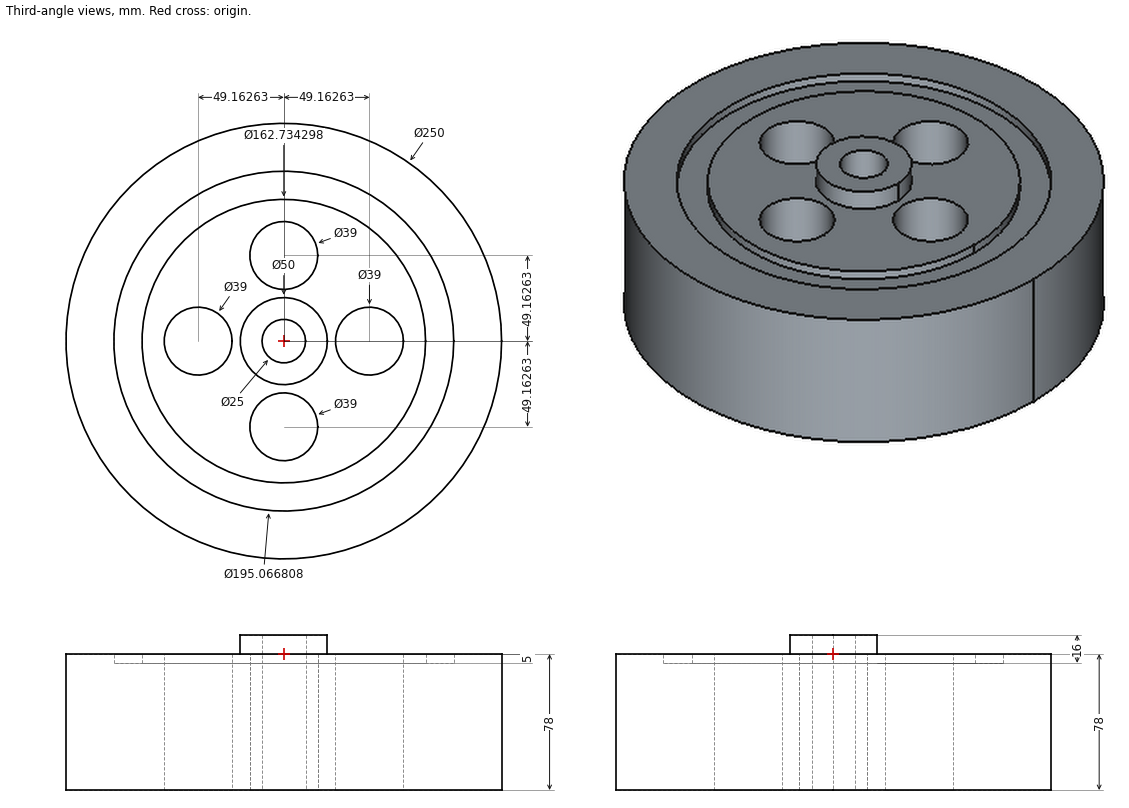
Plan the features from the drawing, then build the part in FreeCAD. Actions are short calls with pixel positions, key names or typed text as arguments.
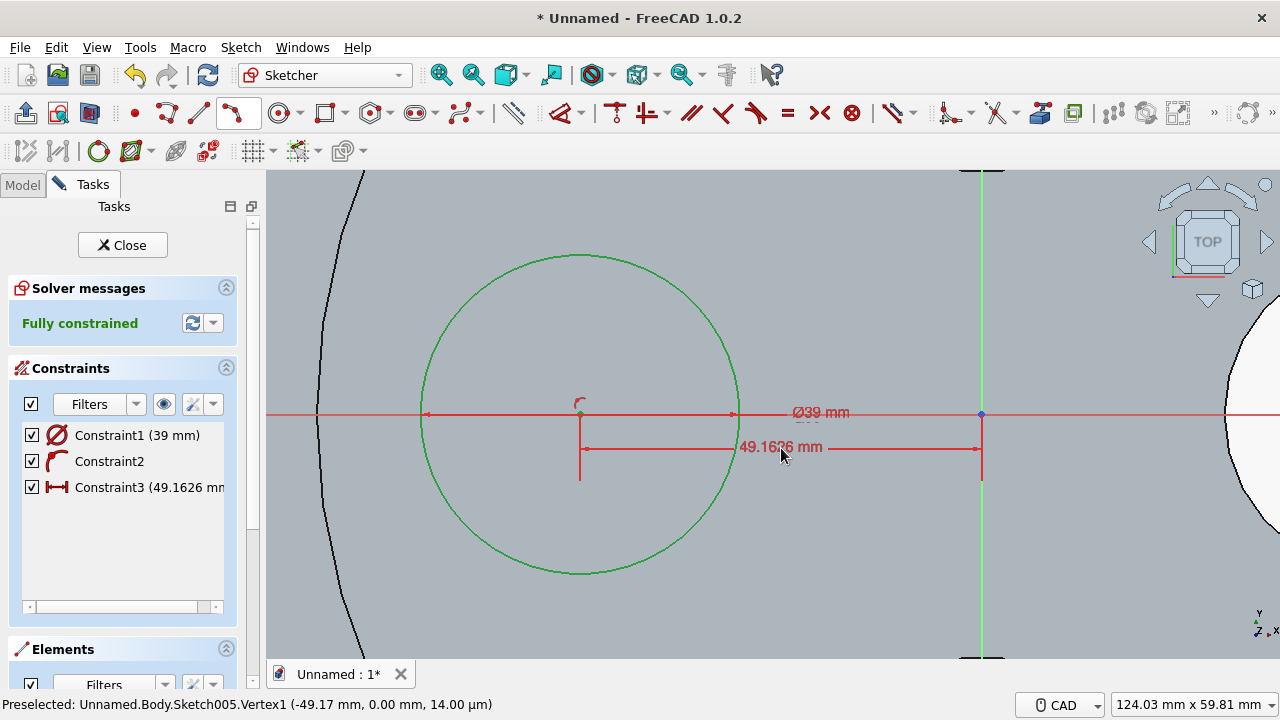
click(123, 245)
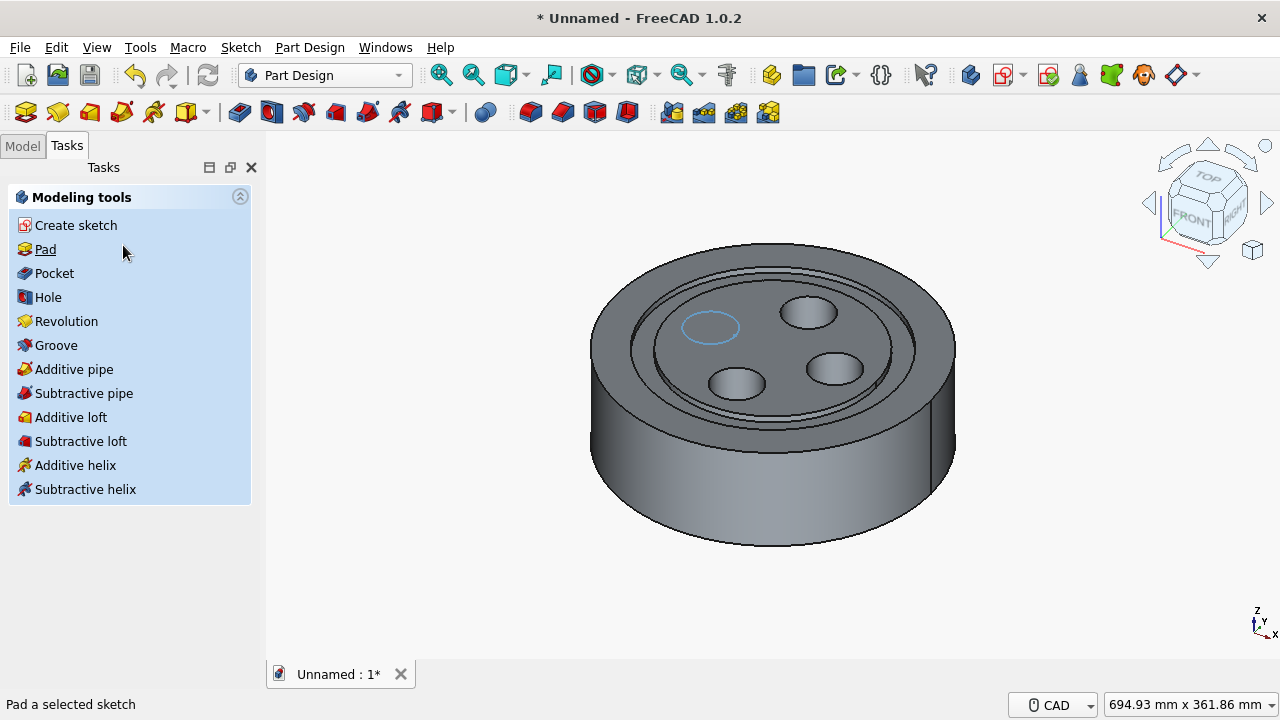
click(240, 112)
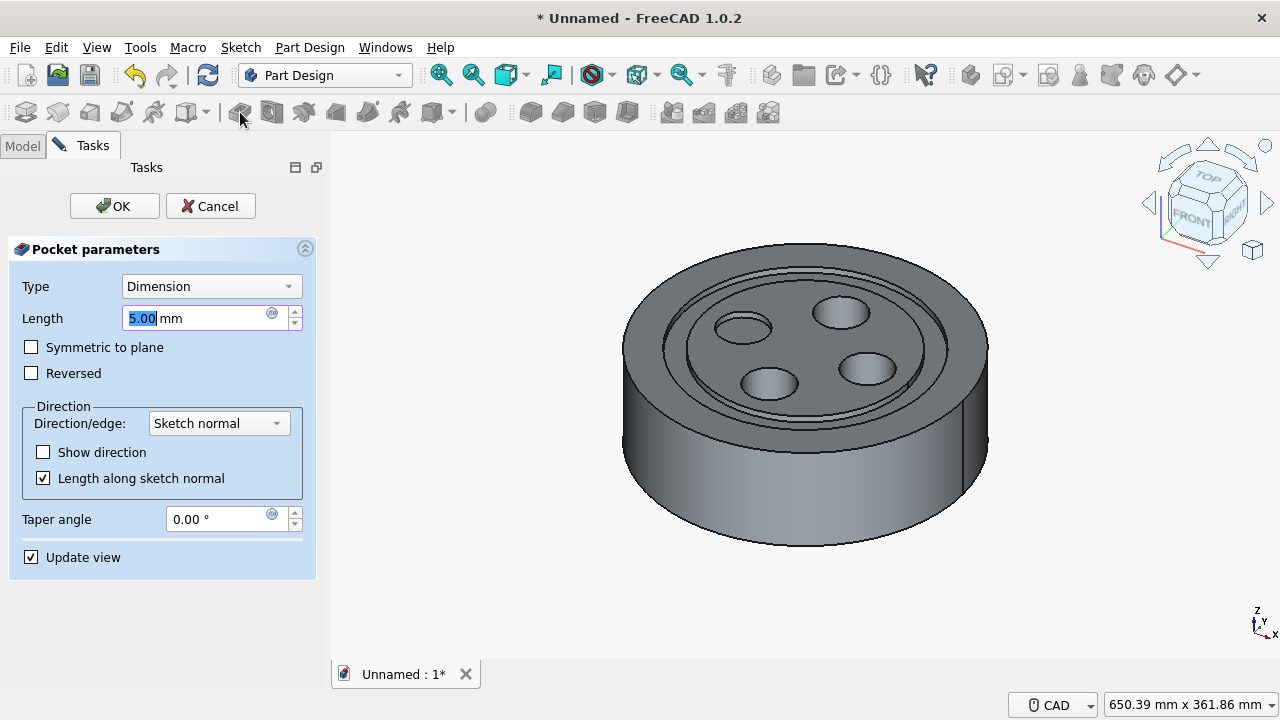
text(78)
key(Tab)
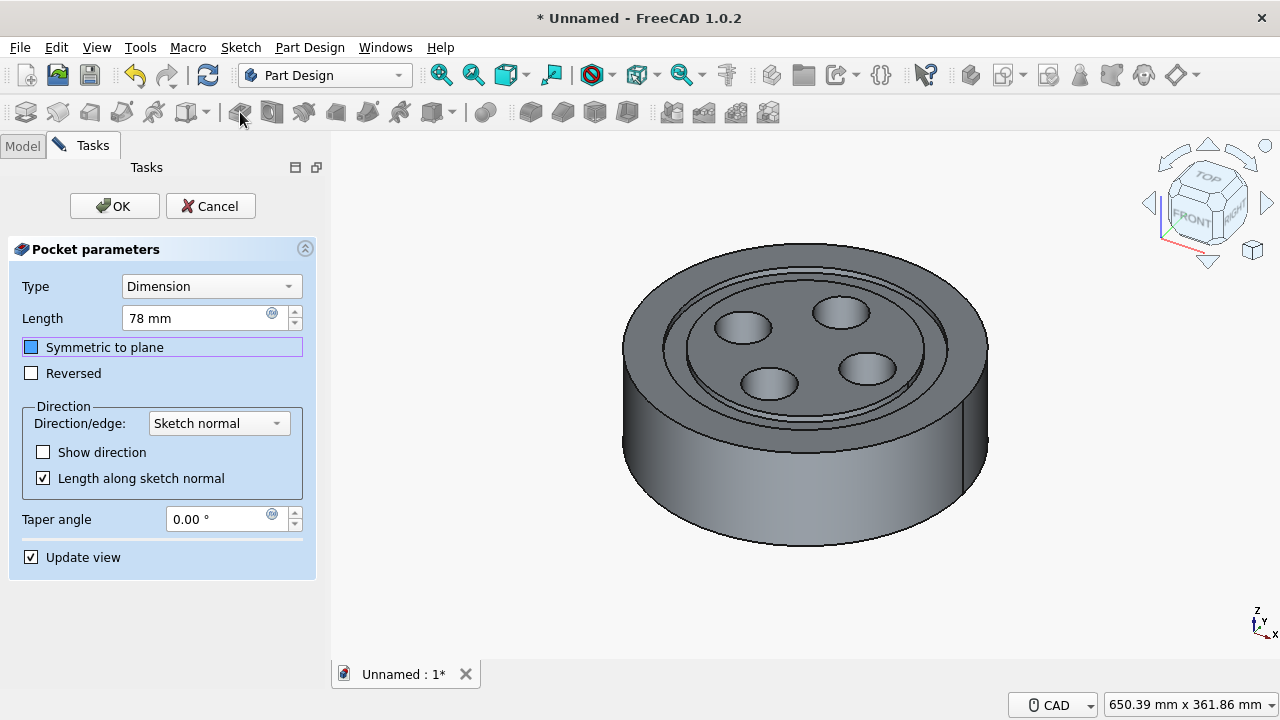
click(115, 206)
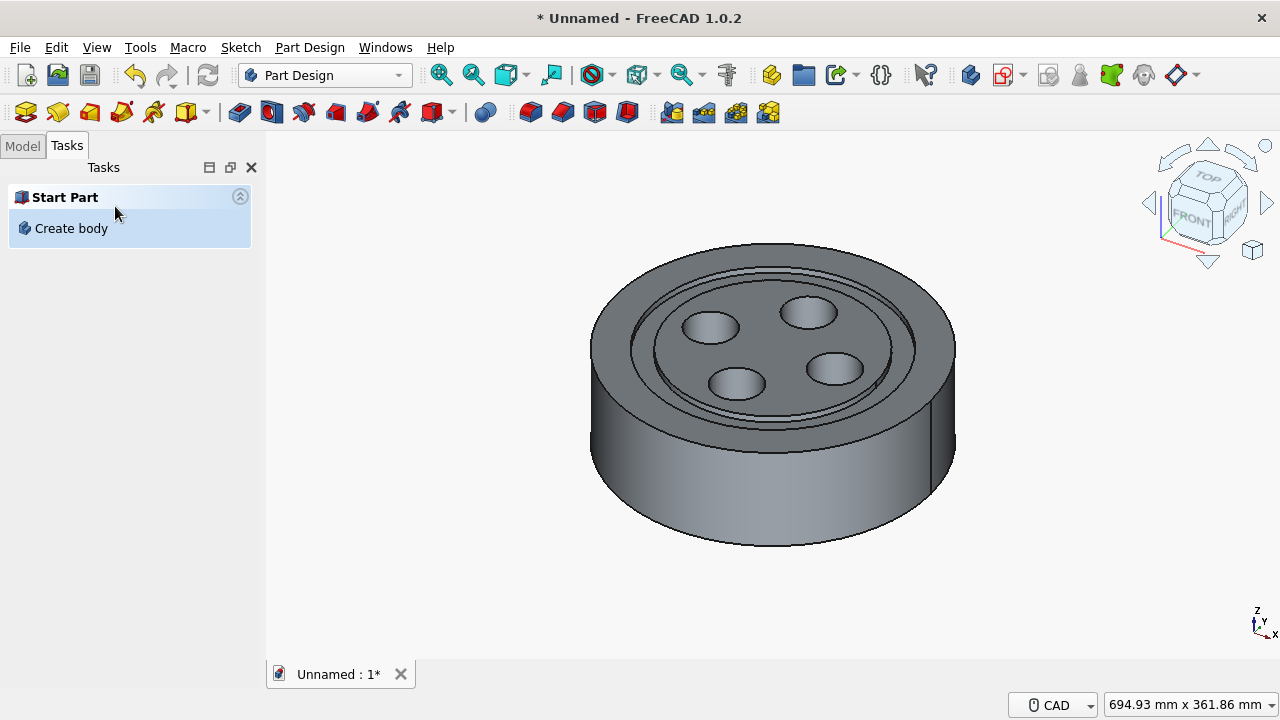
click(899, 368)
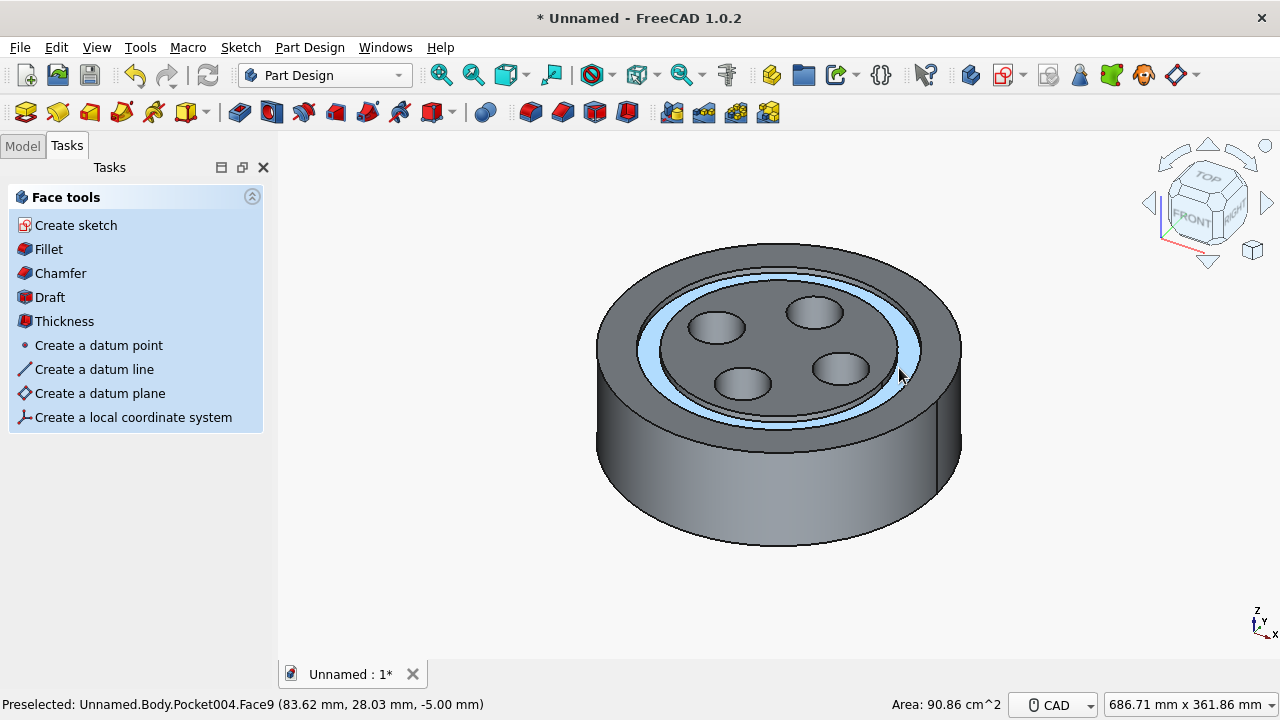
click(1004, 76)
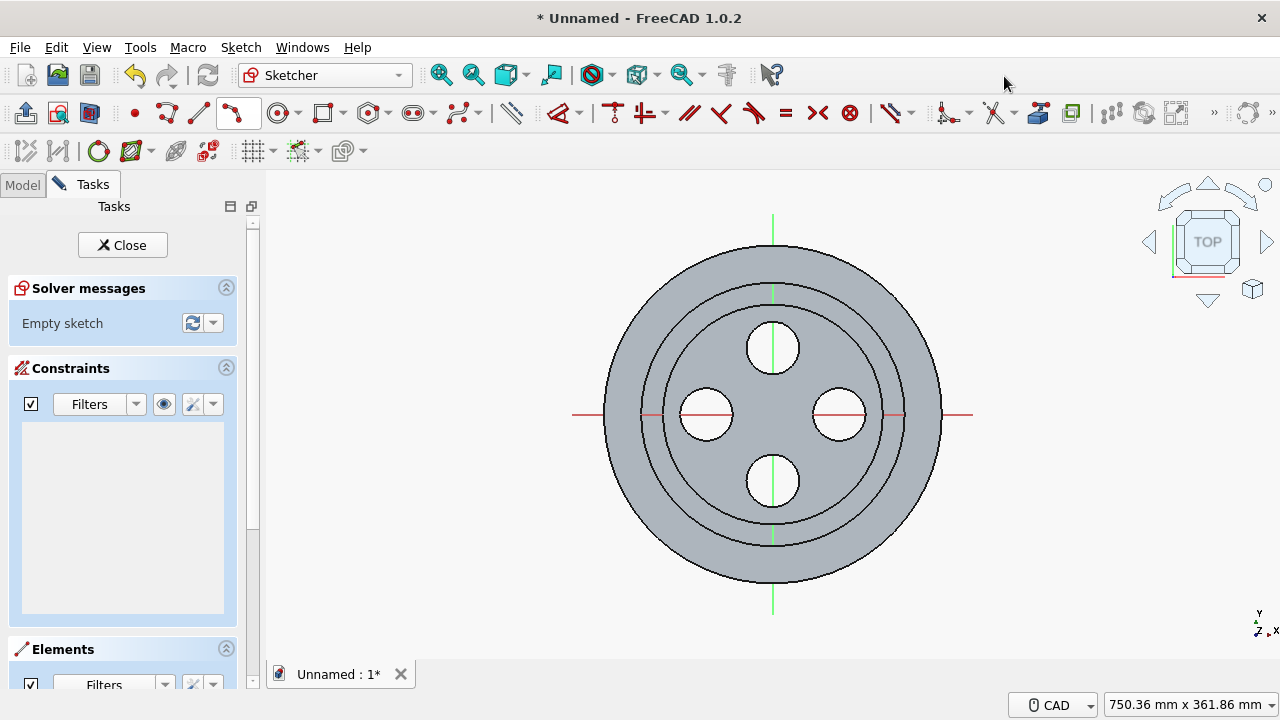
scroll(790, 414, up, 8)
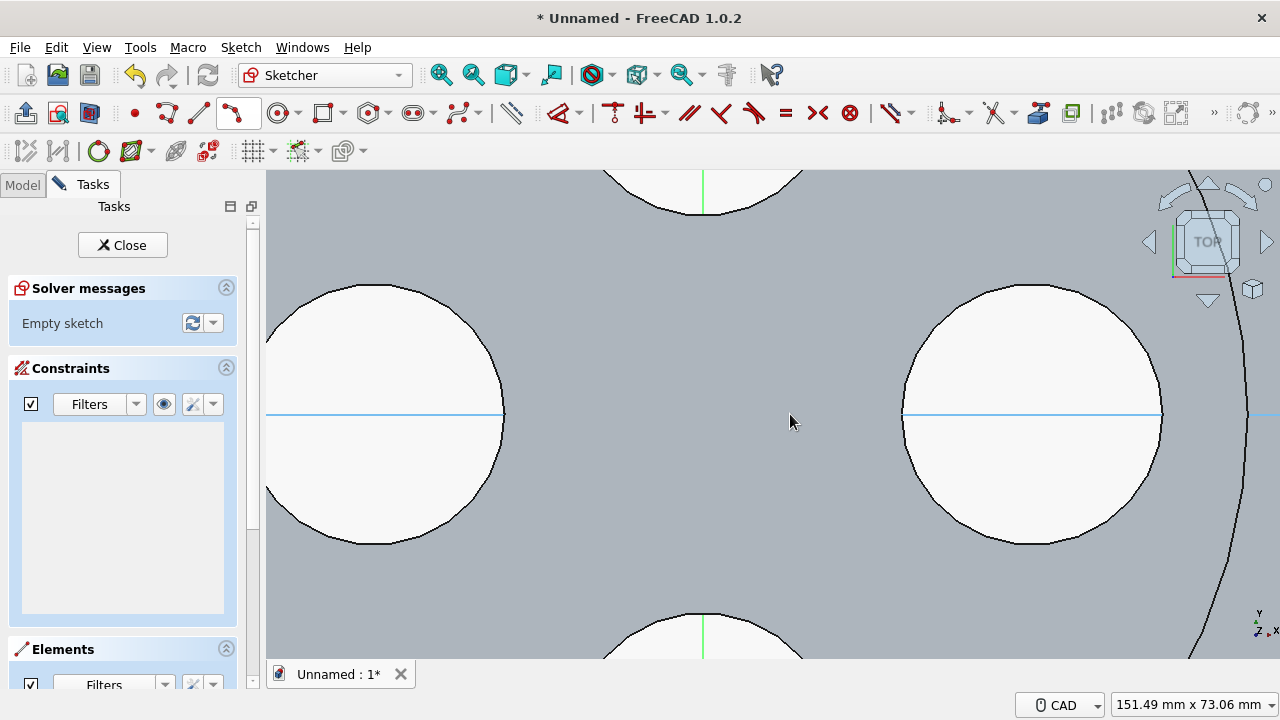
key(g)
key(c)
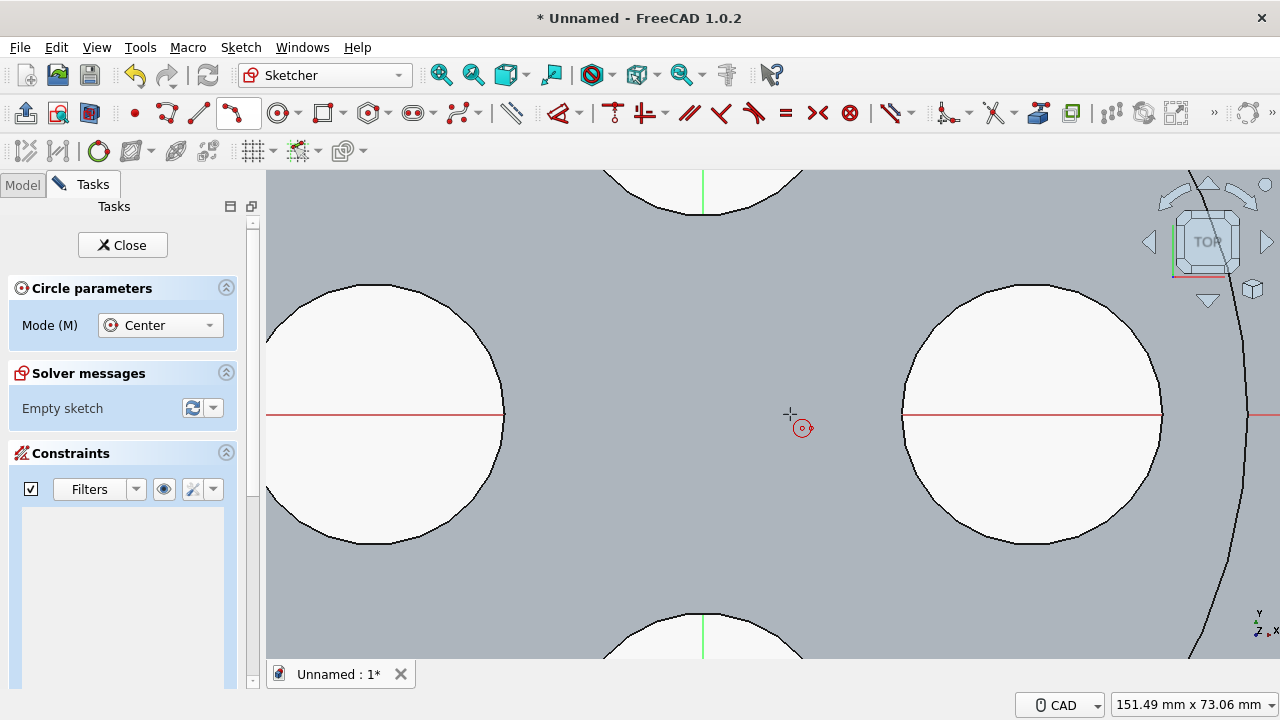
click(703, 414)
move(821, 296)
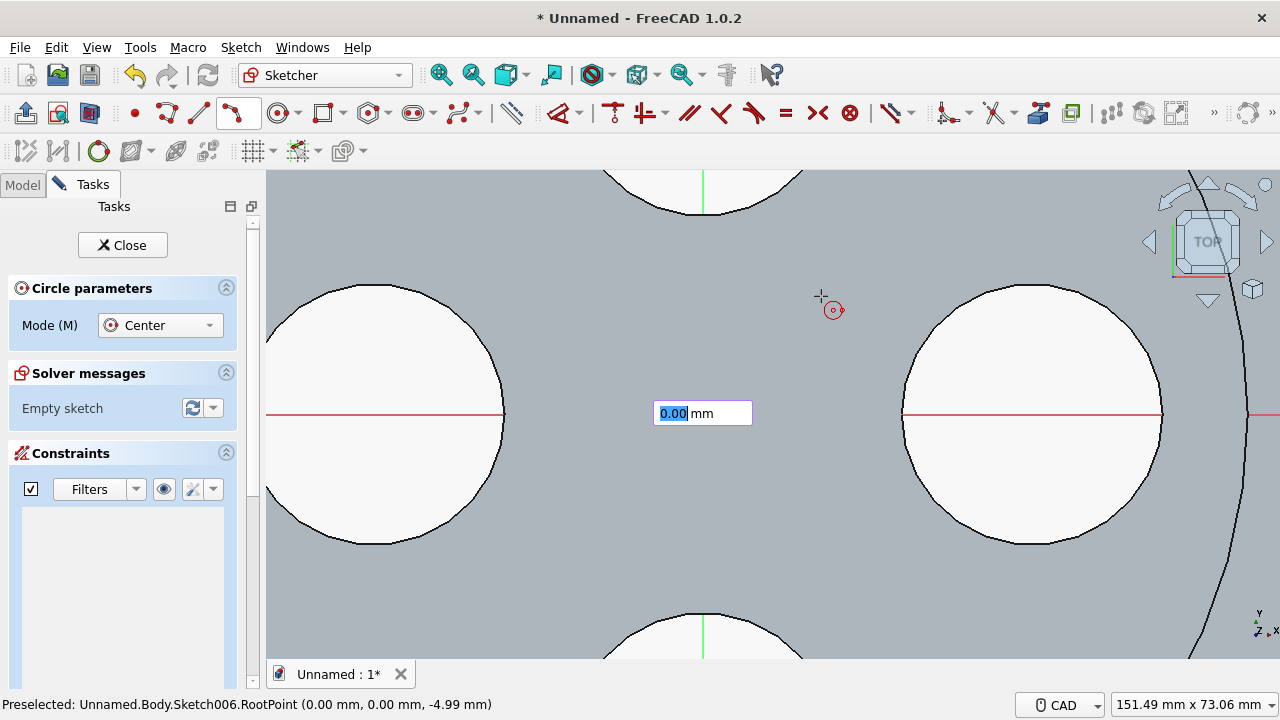
text(50)
key(Return)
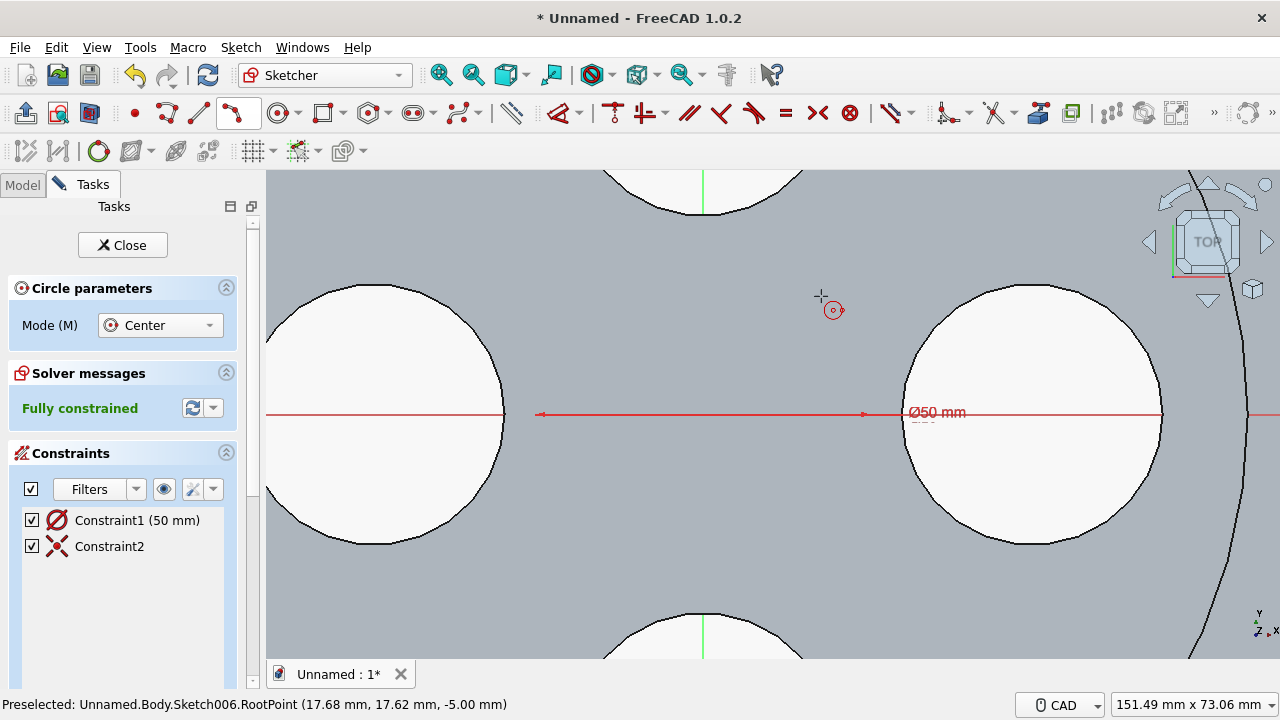
click(703, 414)
move(762, 355)